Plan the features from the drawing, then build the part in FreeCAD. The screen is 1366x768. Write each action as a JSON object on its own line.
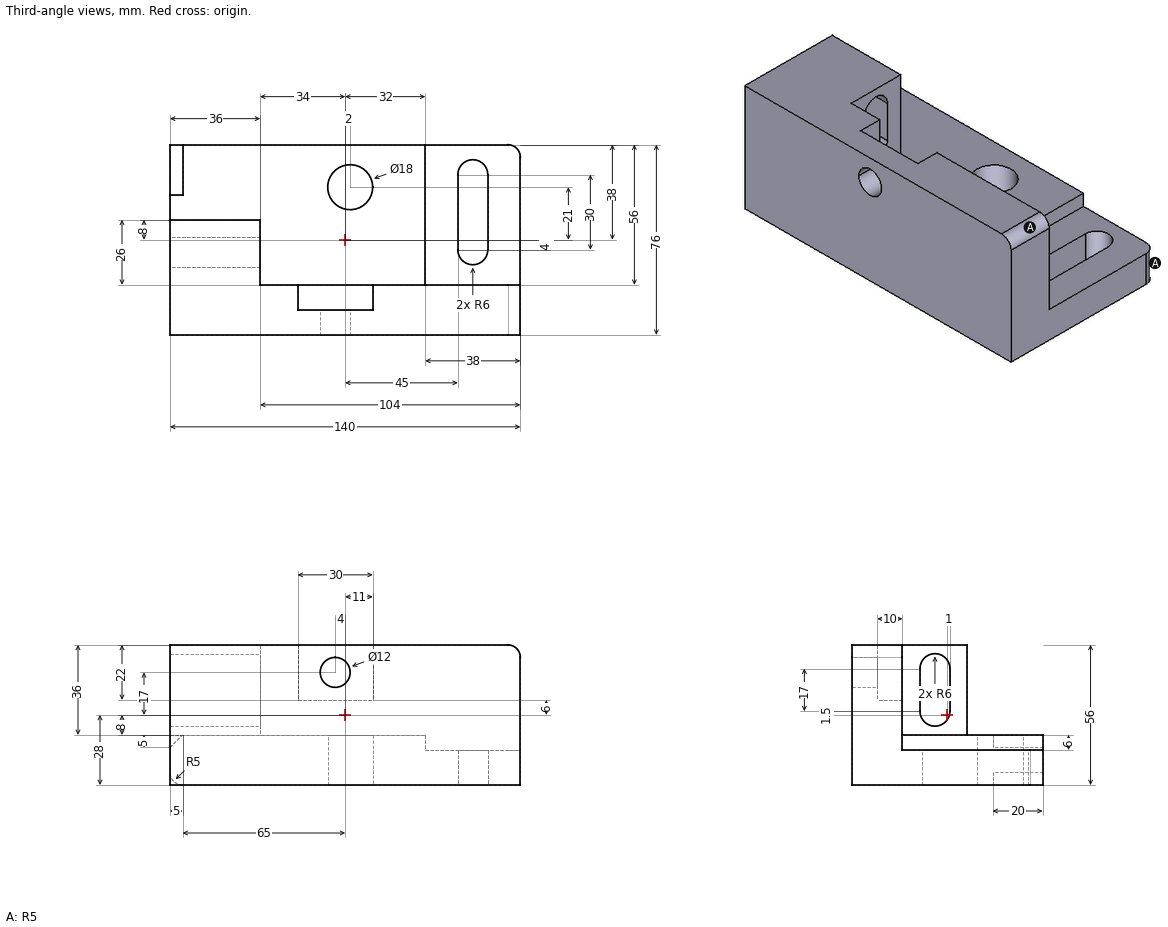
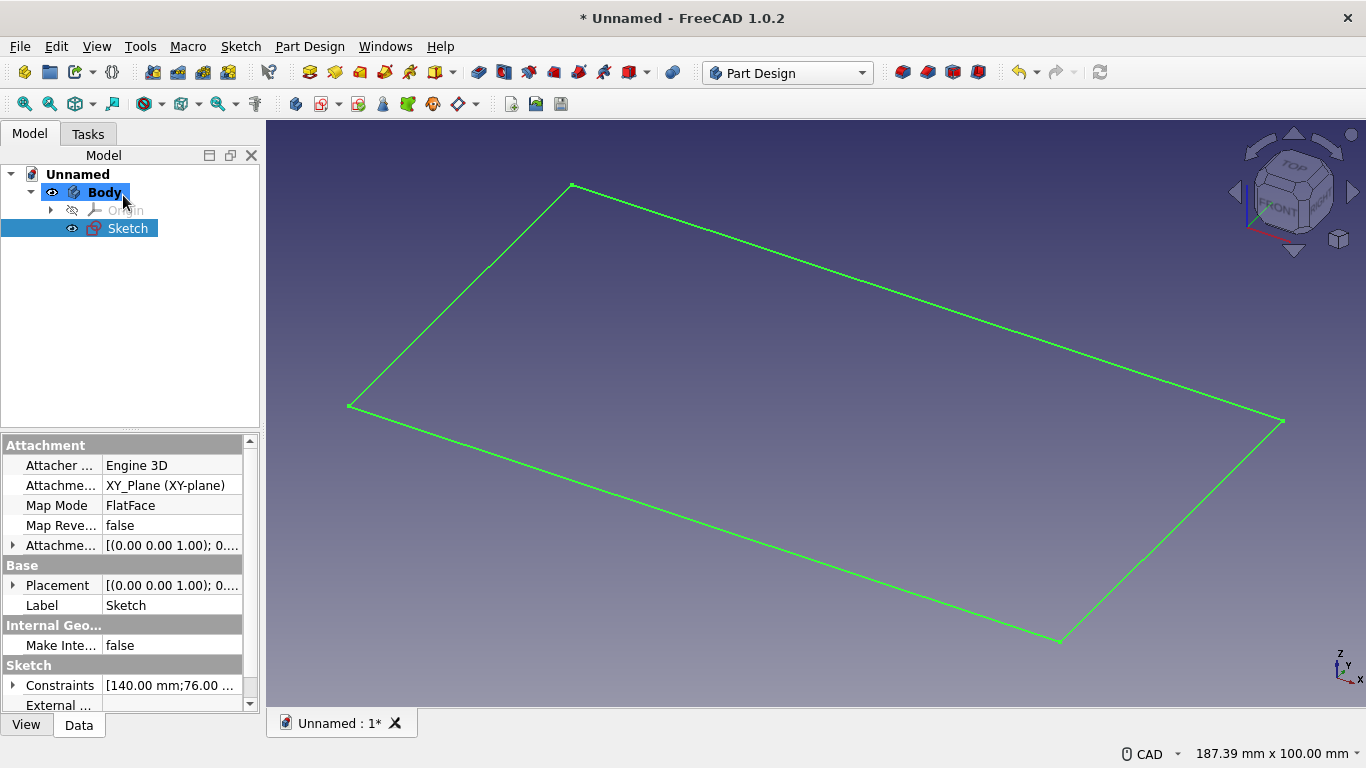
{"action": "left_click", "coordinate": [310, 72]}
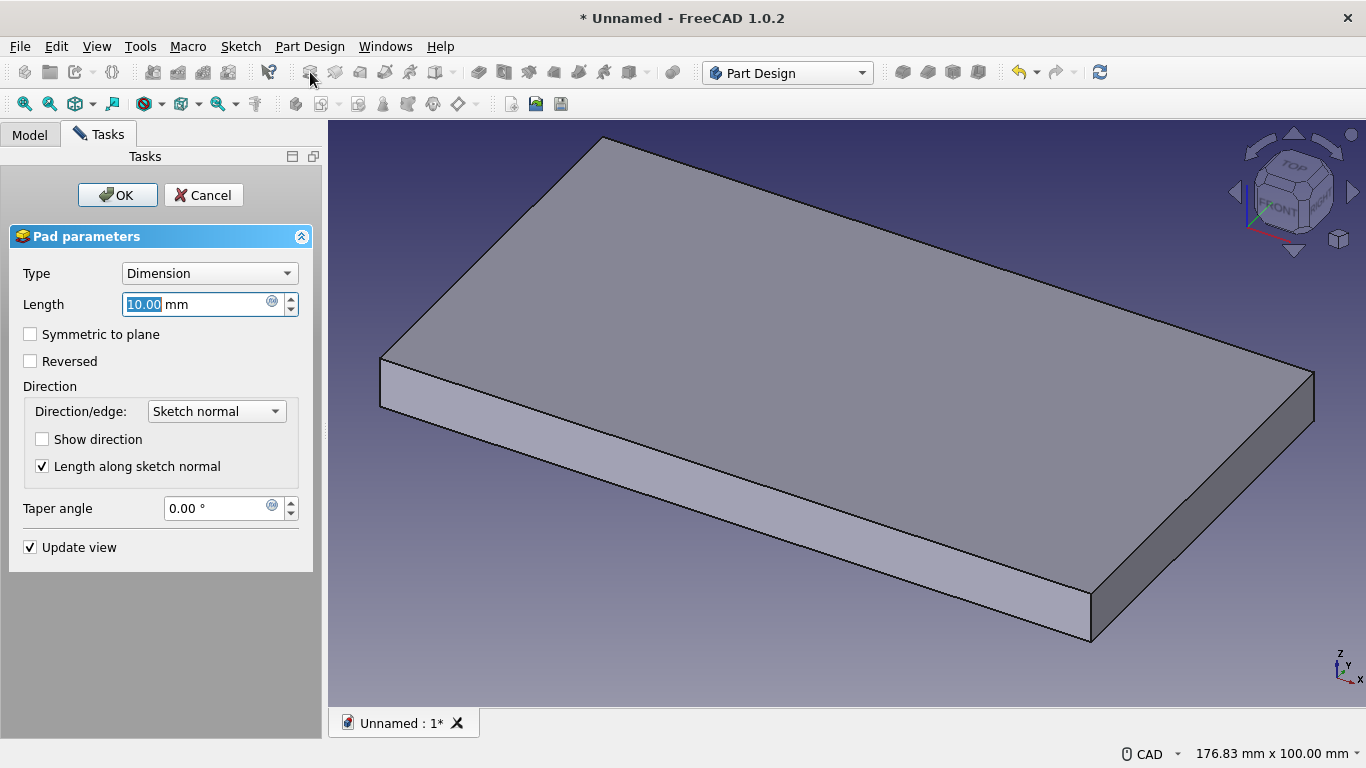
{"action": "type", "text": "56"}
{"action": "key", "text": "Tab"}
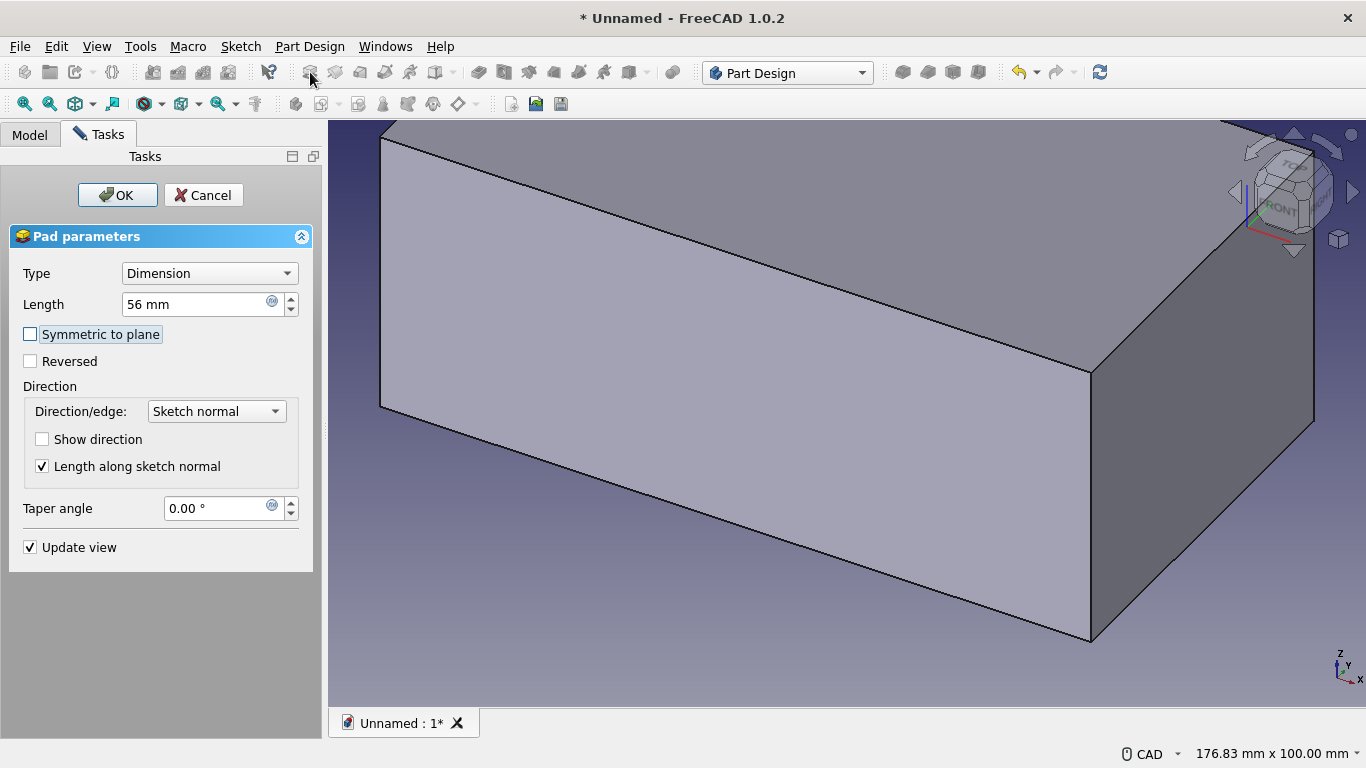
{"action": "left_click", "coordinate": [31, 334]}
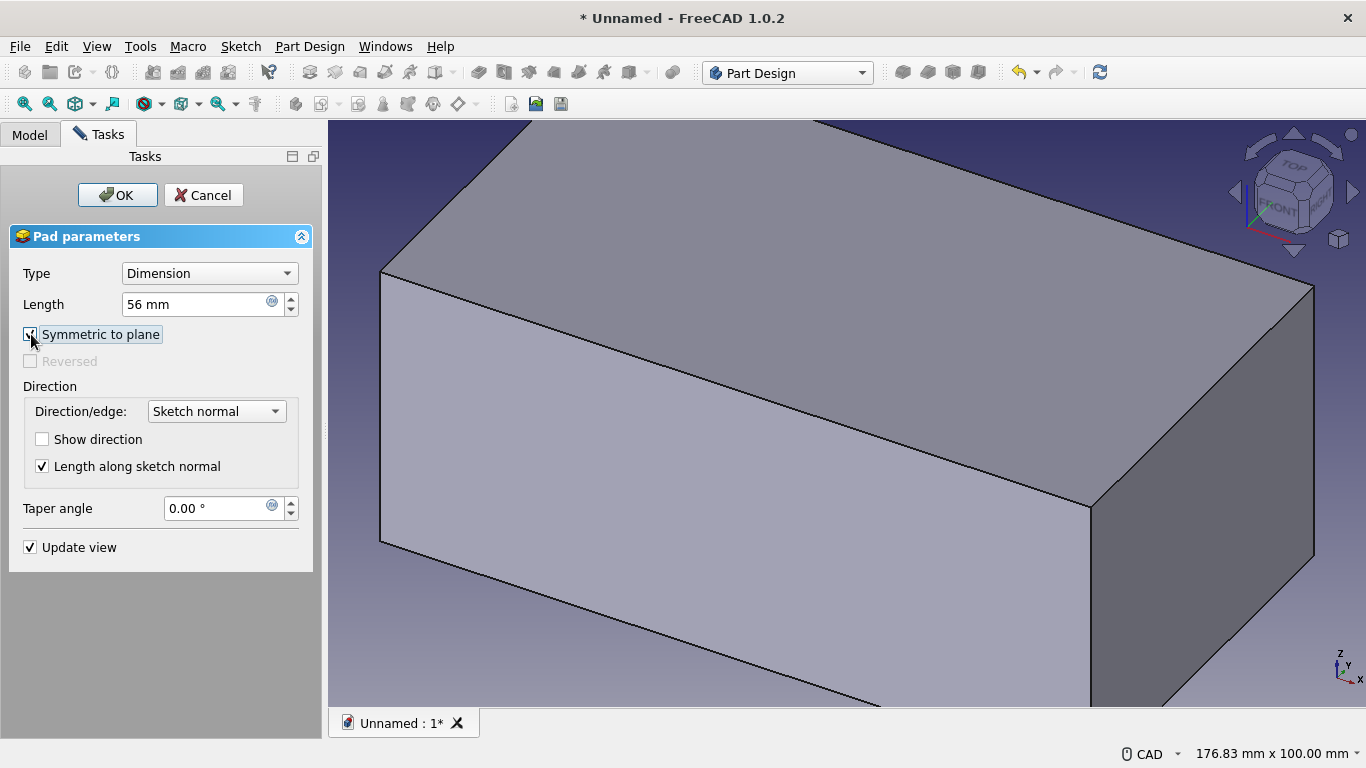
{"action": "left_click", "coordinate": [118, 195]}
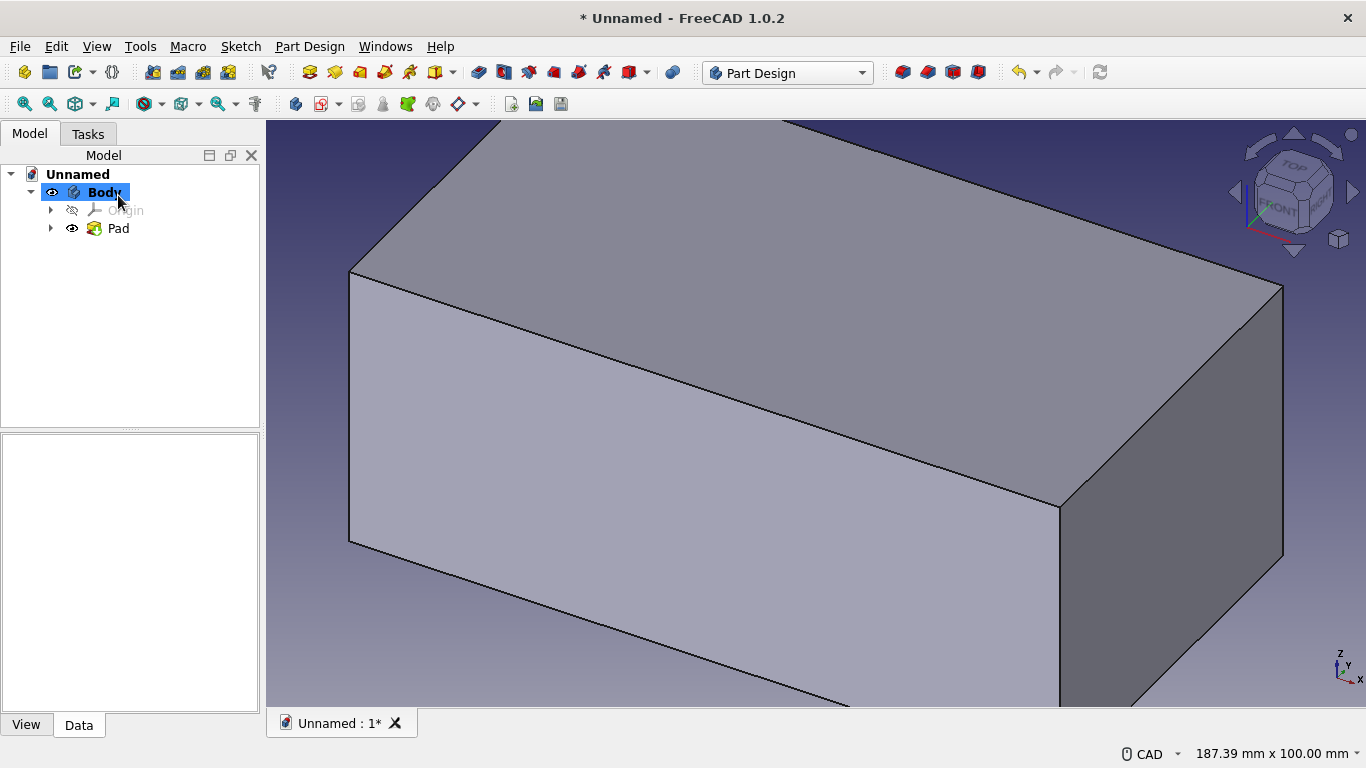
{"action": "key", "text": "v f"}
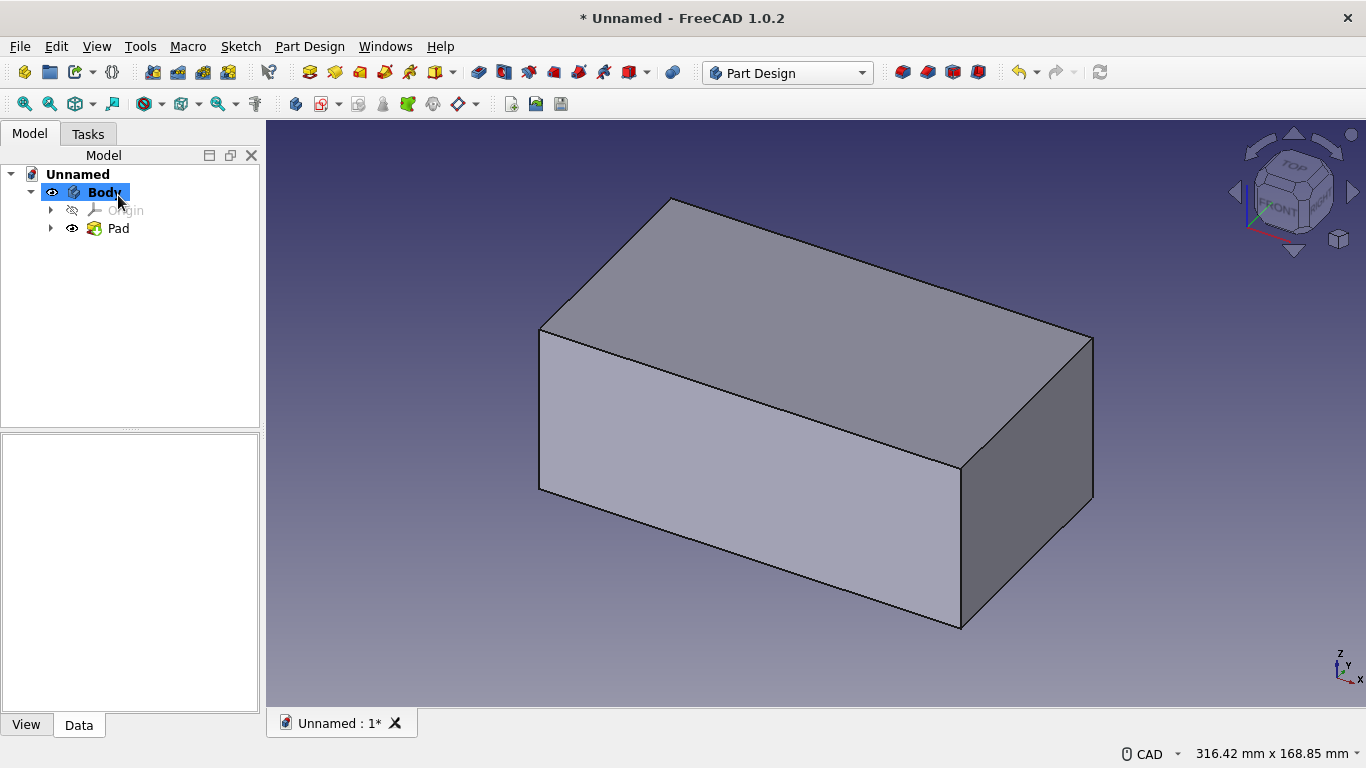
{"action": "left_click", "coordinate": [876, 353]}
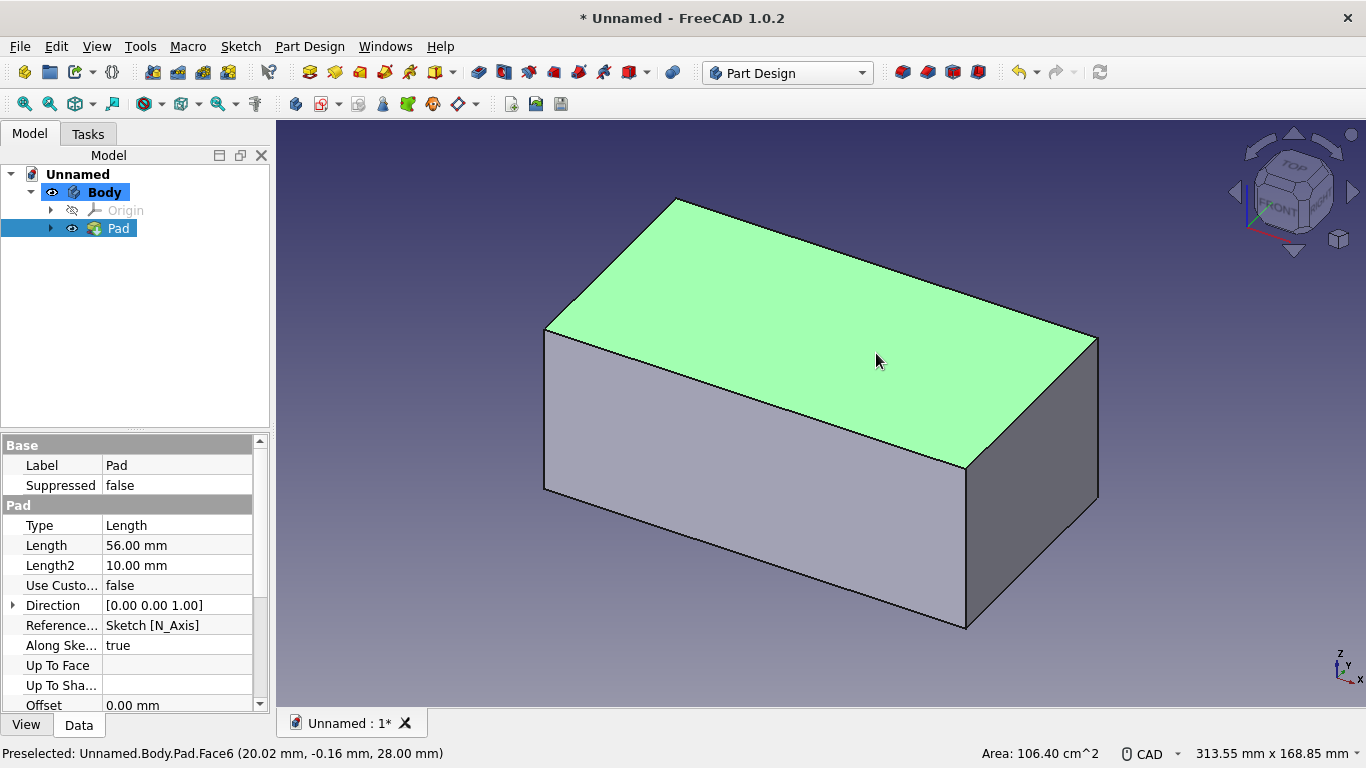
{"action": "left_click", "coordinate": [320, 104]}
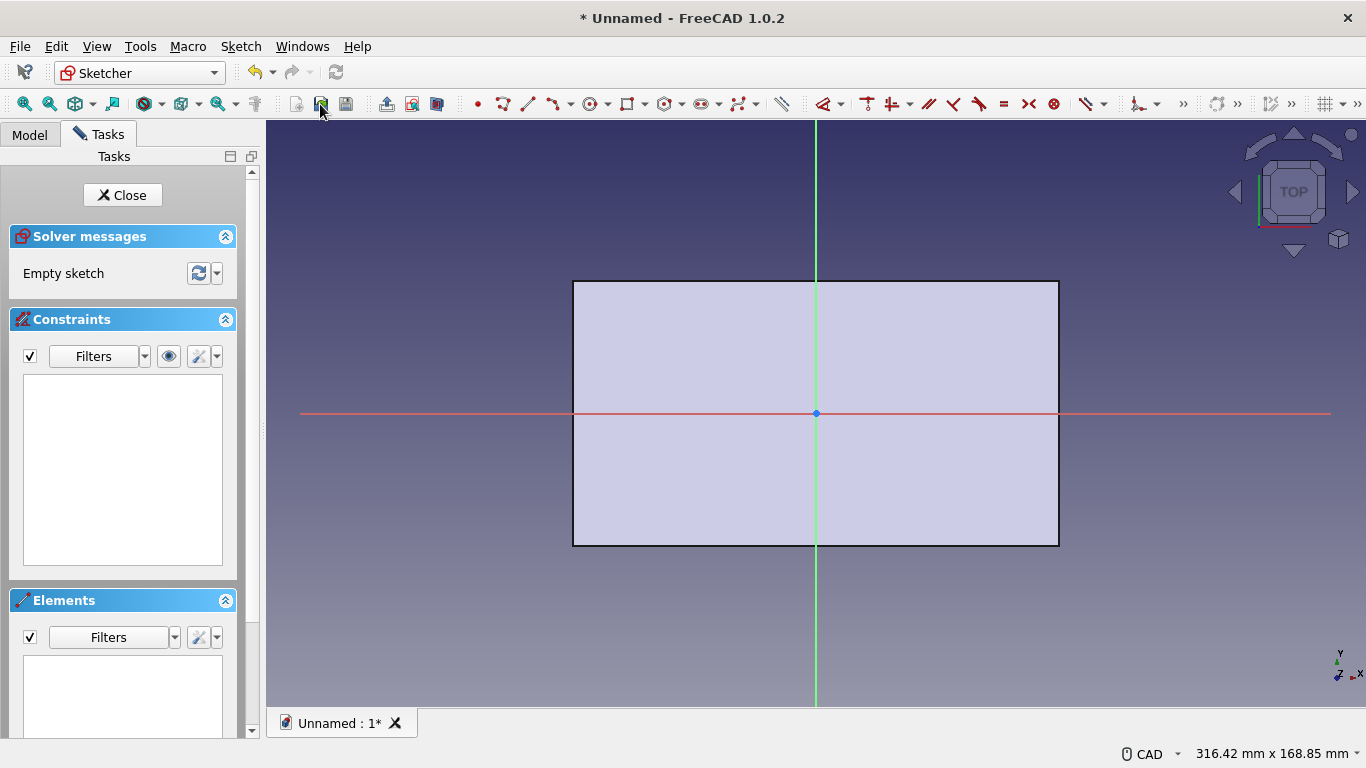
{"action": "left_click", "coordinate": [503, 104]}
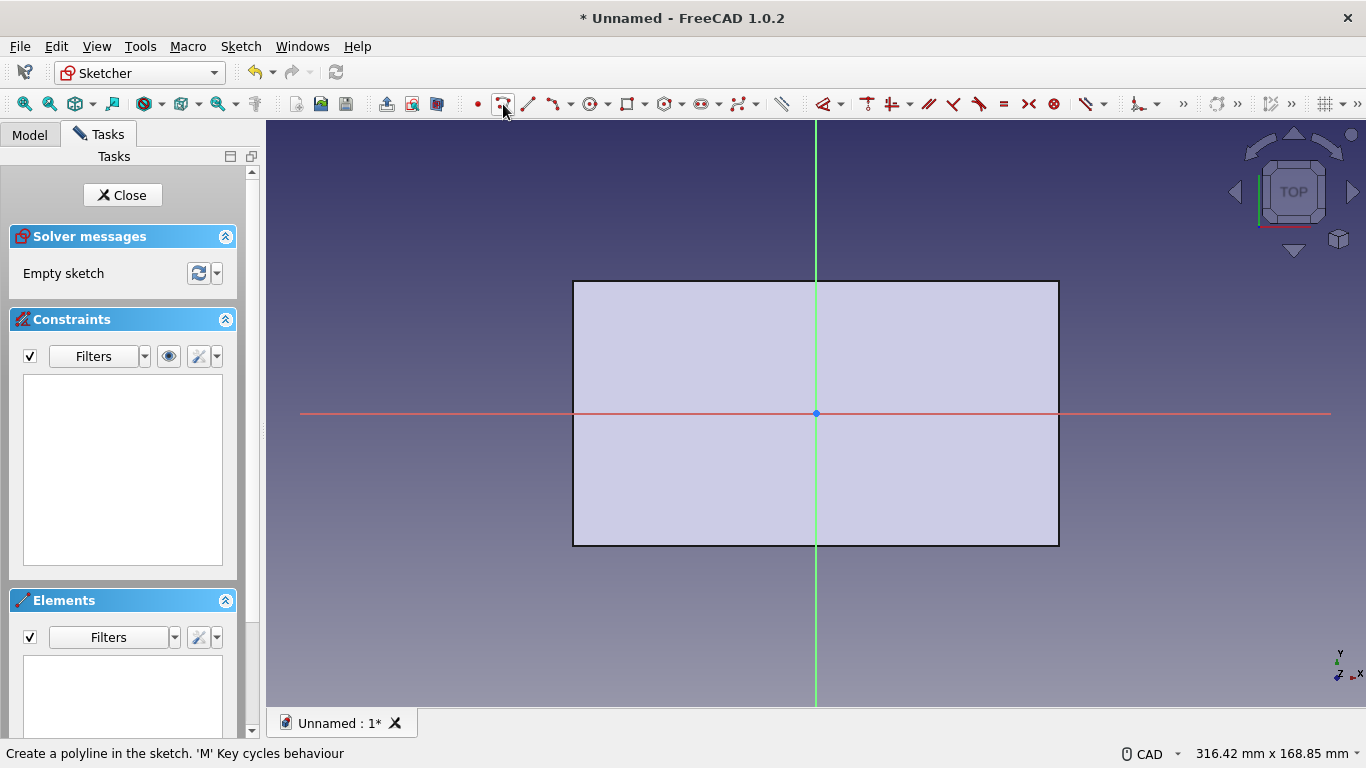
{"action": "left_click", "coordinate": [698, 386]}
{"action": "left_click", "coordinate": [698, 476]}
{"action": "left_click", "coordinate": [1059, 476]}
{"action": "left_click", "coordinate": [1059, 281]}
{"action": "left_click", "coordinate": [573, 281]}
{"action": "left_click", "coordinate": [573, 386]}
{"action": "left_click", "coordinate": [698, 387]}
{"action": "key", "text": "Escape"}
{"action": "key", "text": "Escape"}